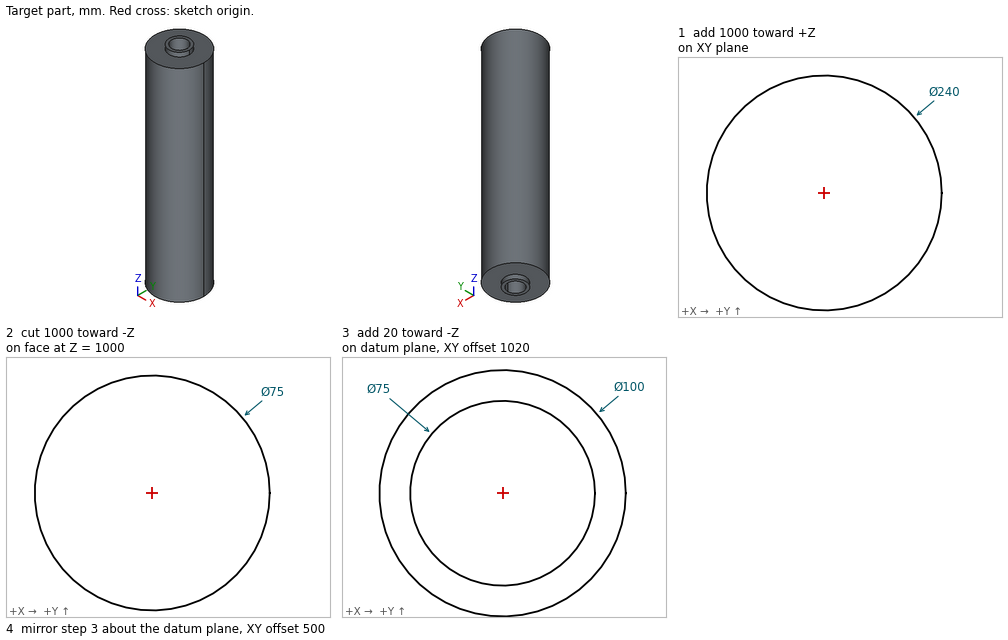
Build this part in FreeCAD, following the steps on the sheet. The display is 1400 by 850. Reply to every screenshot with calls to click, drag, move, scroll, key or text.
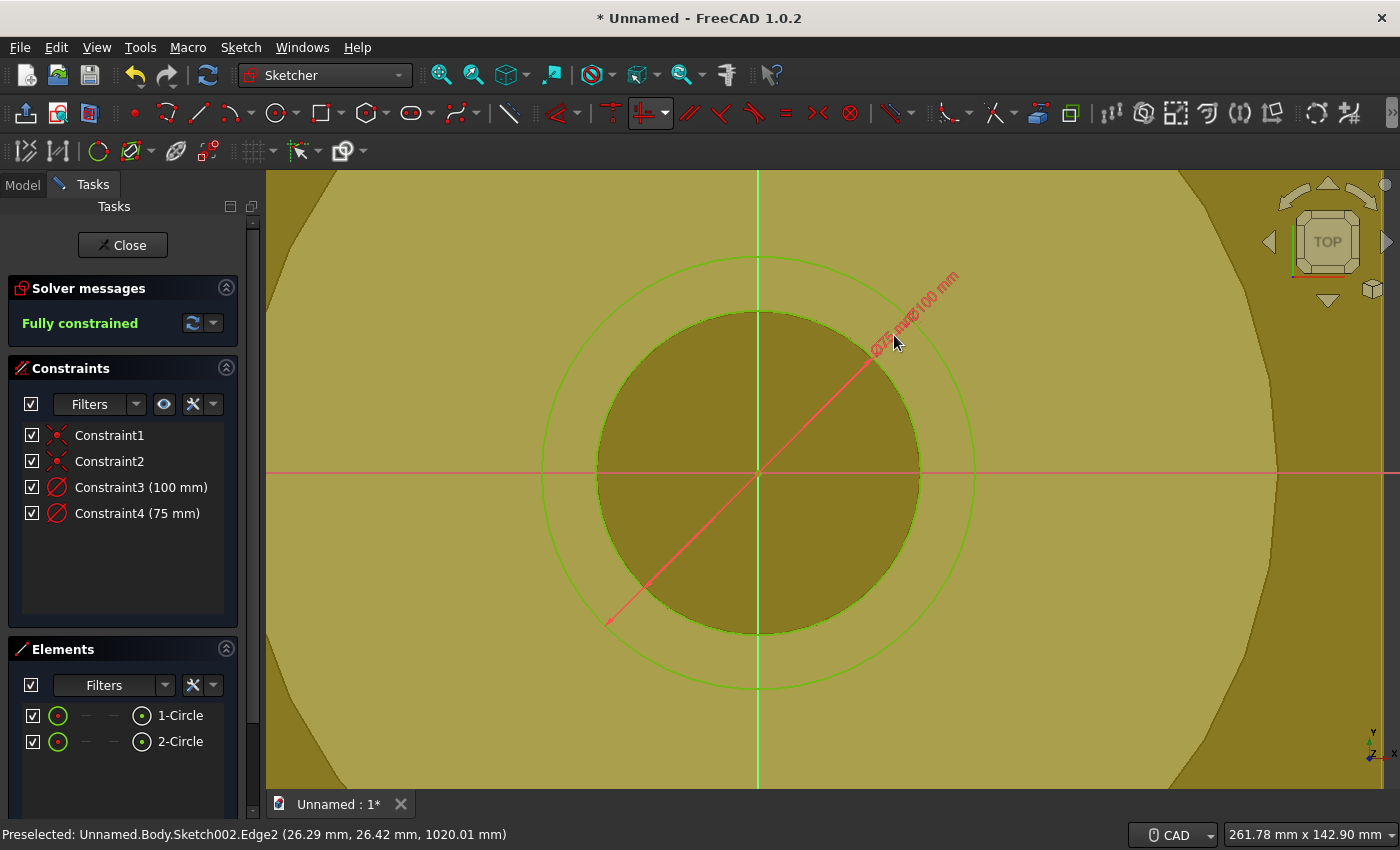
click(123, 245)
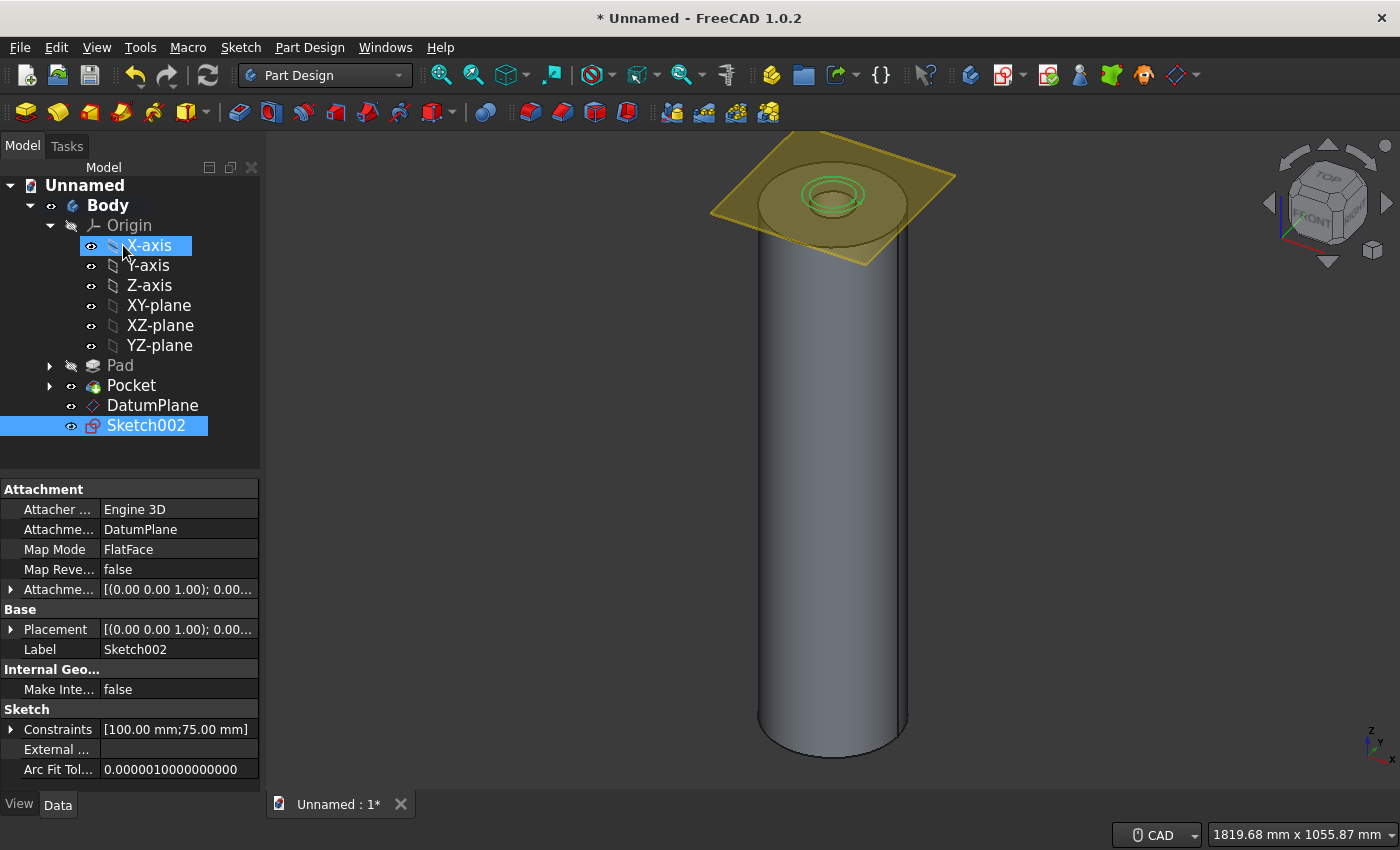
click(26, 112)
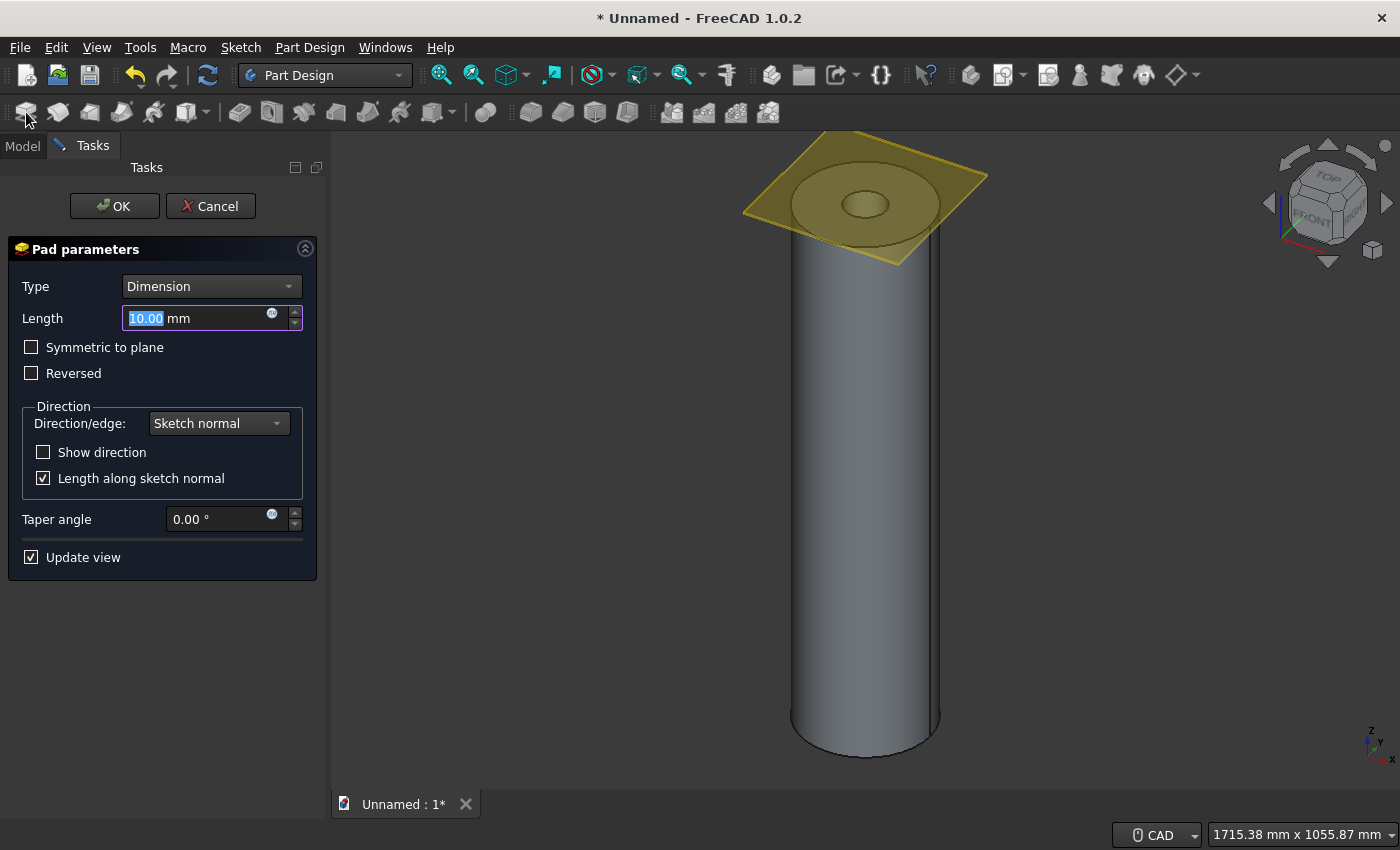
text(20)
key(Tab)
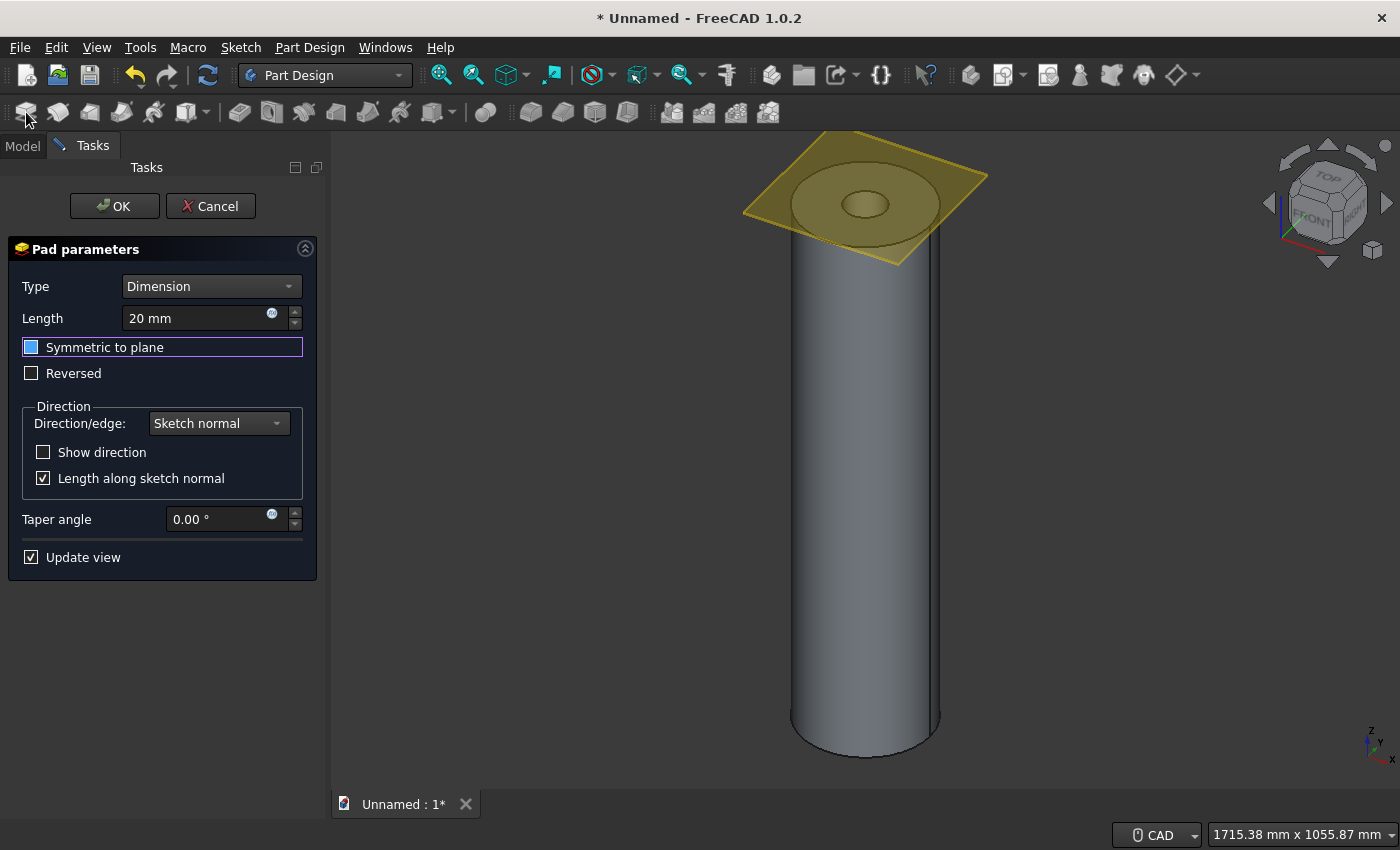
click(30, 373)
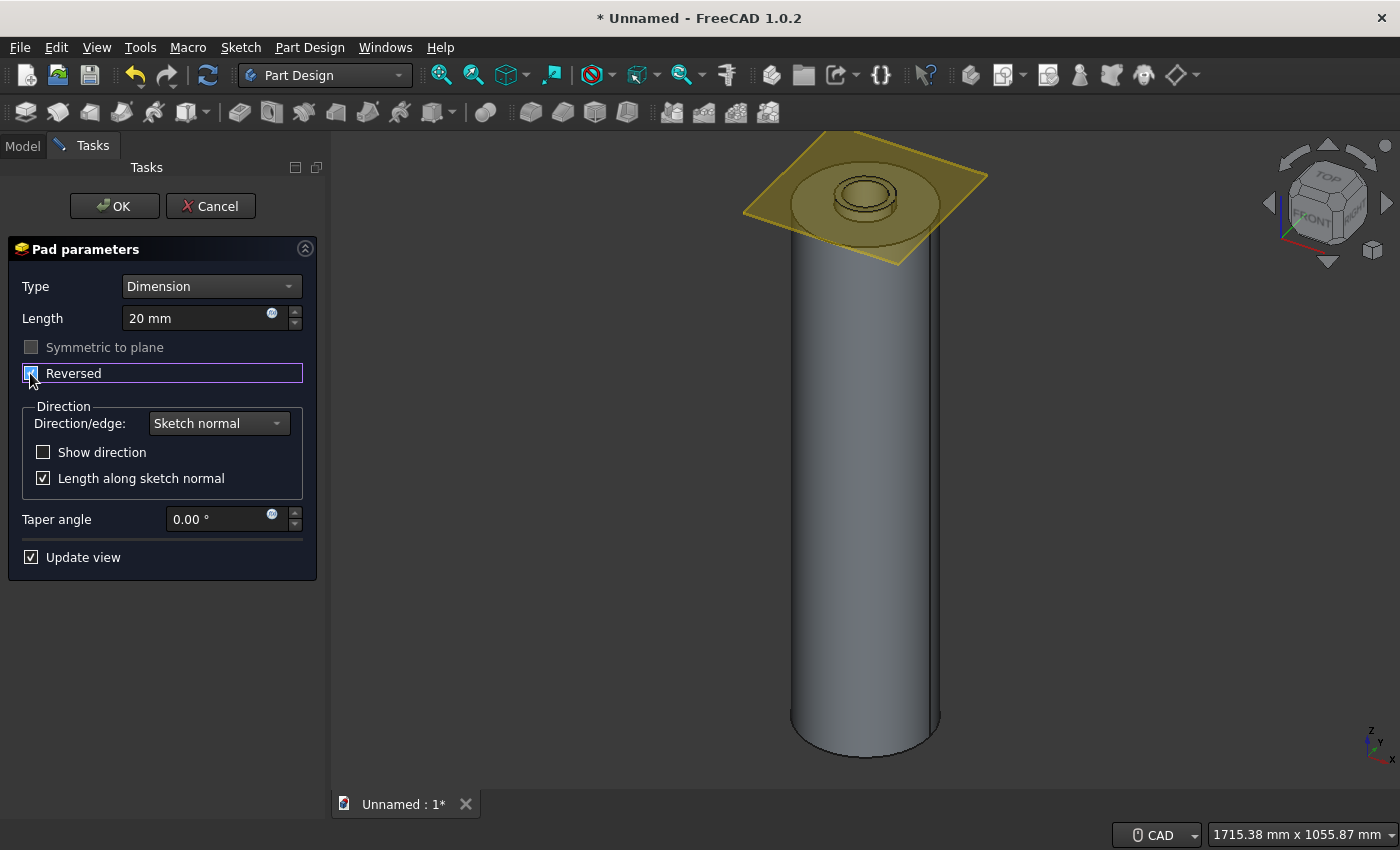
click(115, 206)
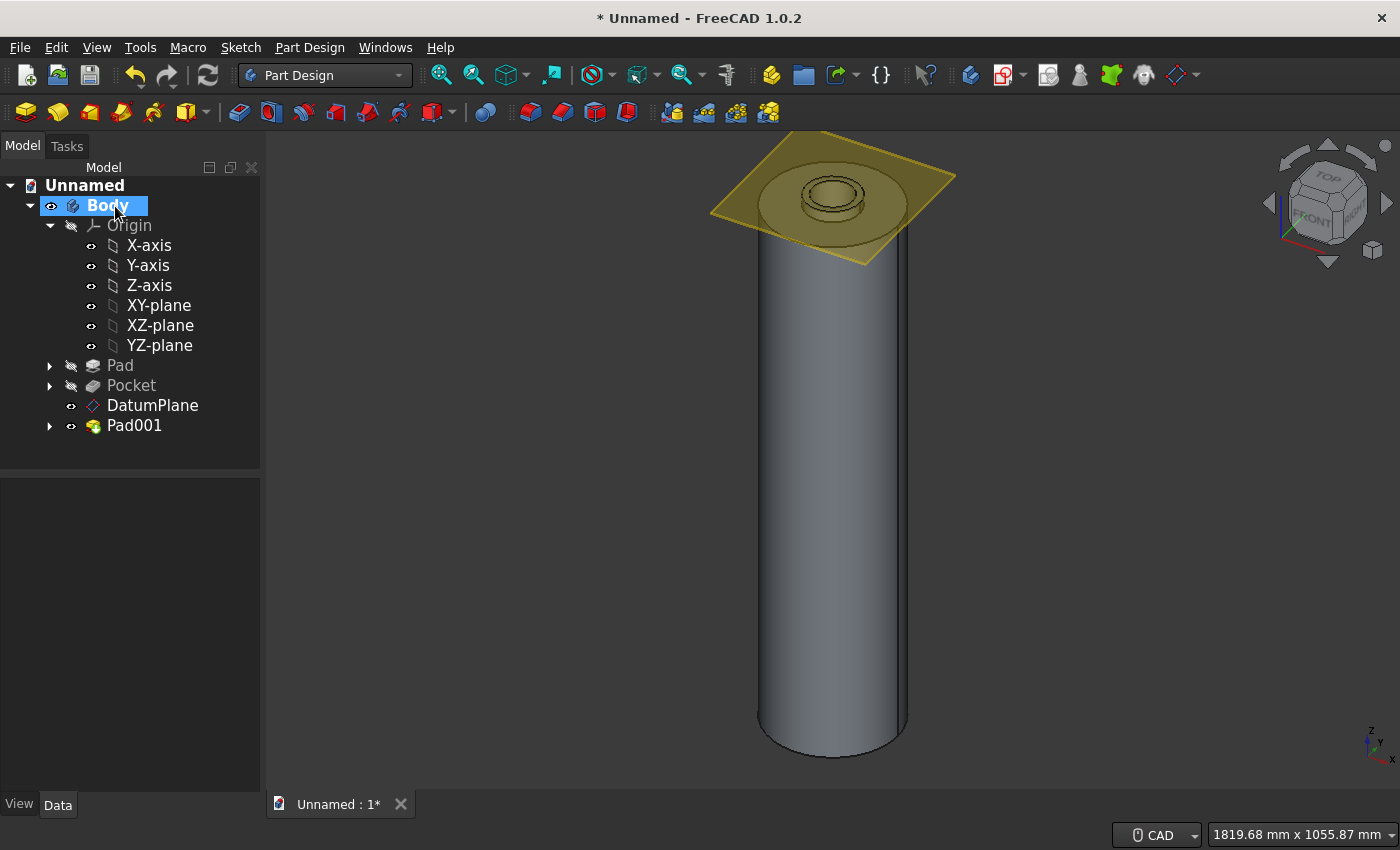
click(116, 406)
key(space)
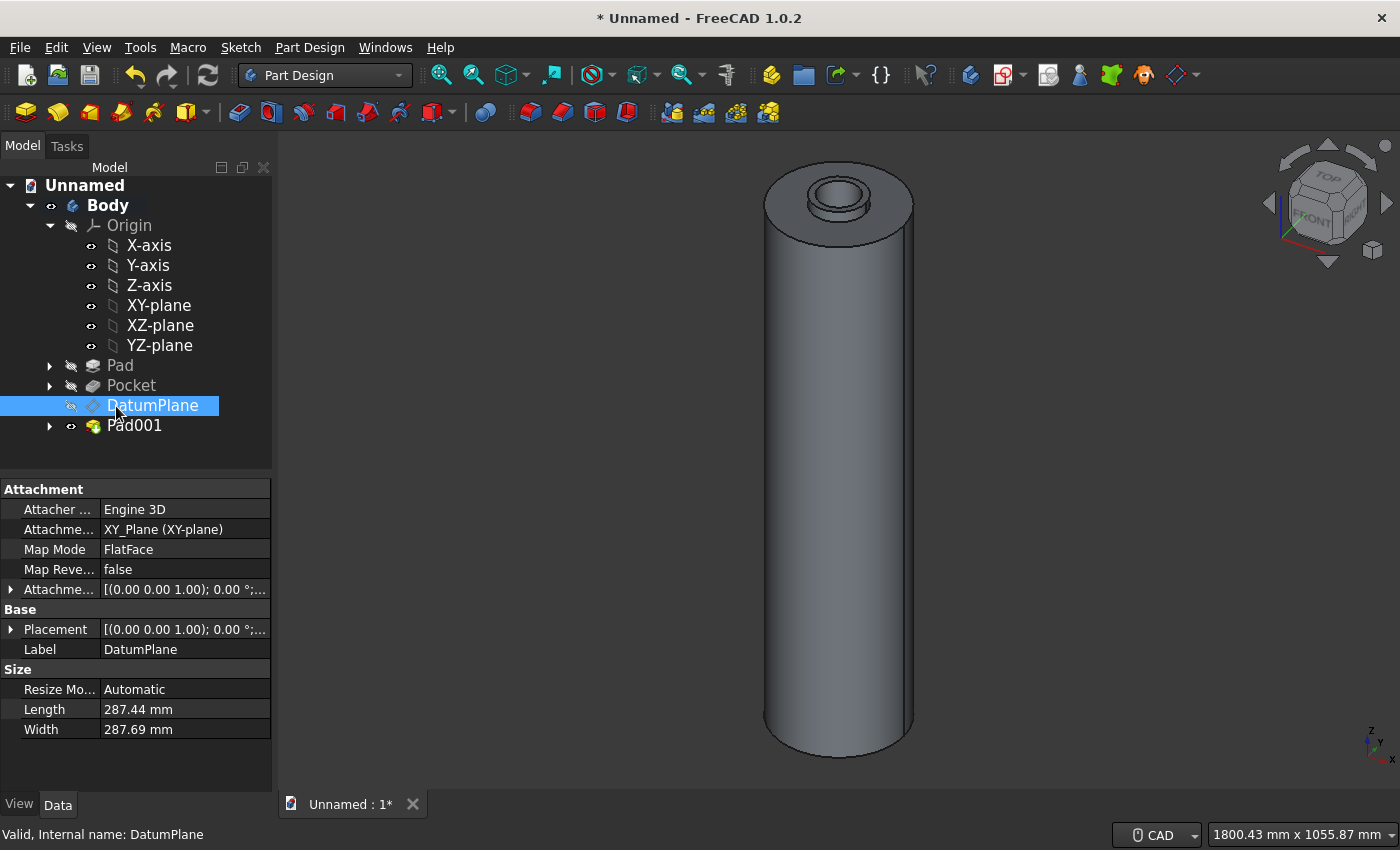
click(136, 306)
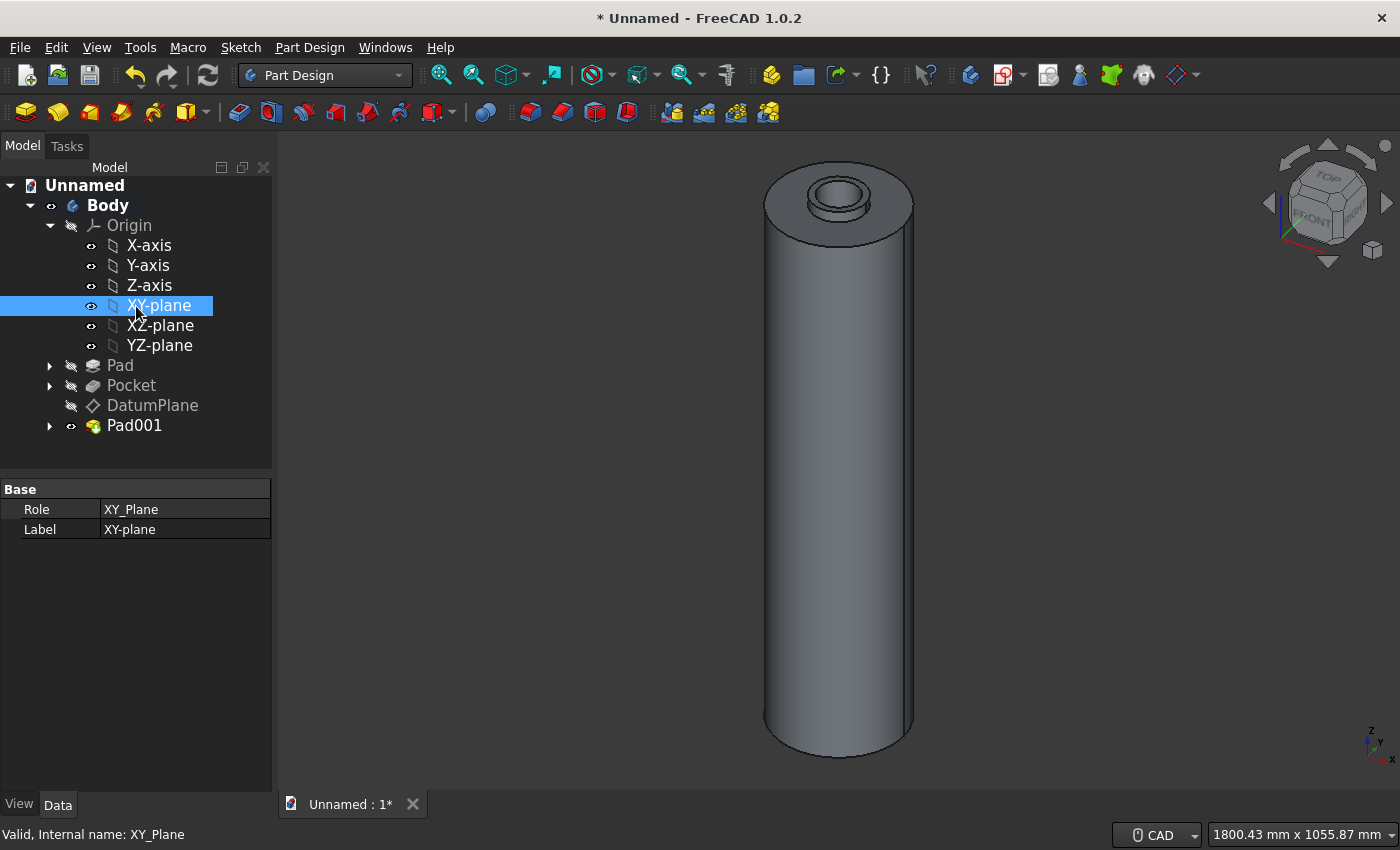
click(1176, 76)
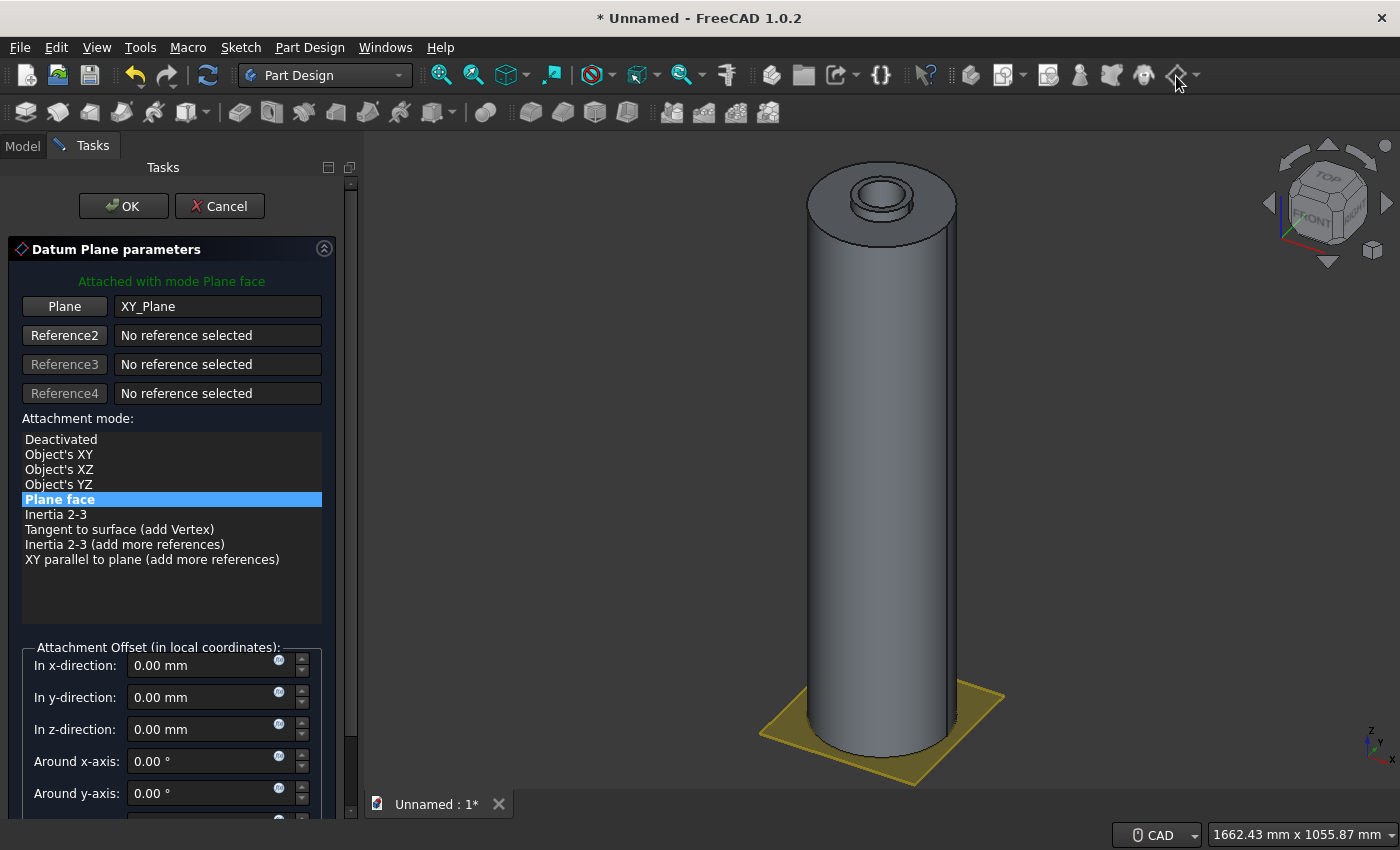
triple_click(210, 729)